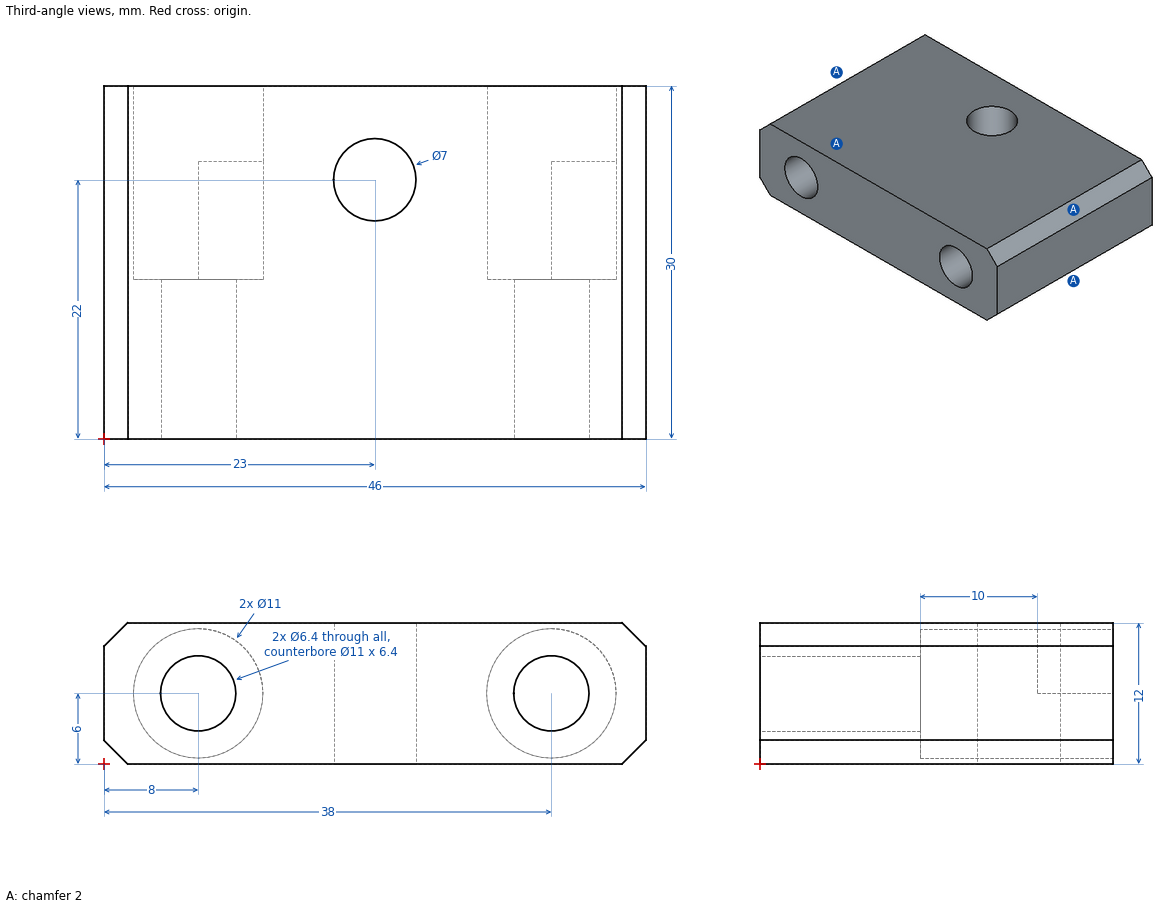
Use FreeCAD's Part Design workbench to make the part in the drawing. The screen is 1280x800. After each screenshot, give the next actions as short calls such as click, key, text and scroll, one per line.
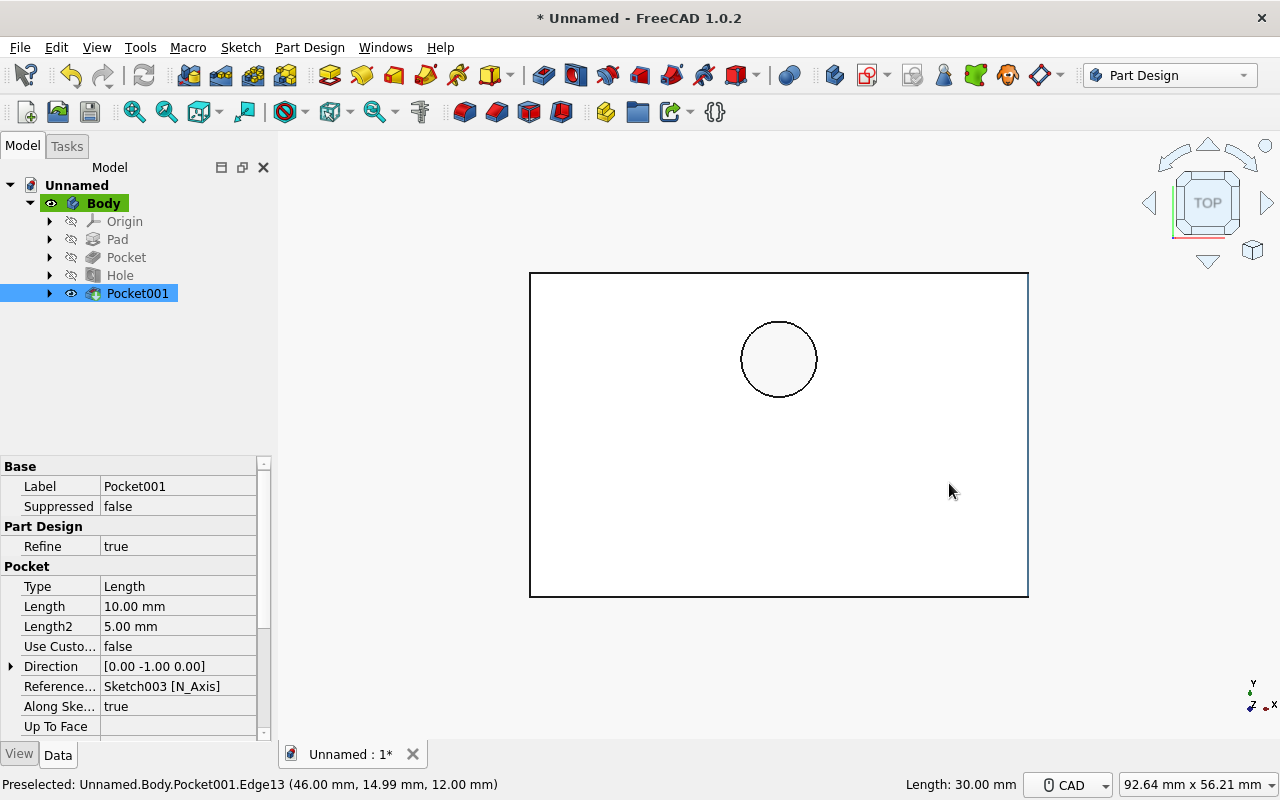
click(530, 434, ctrl)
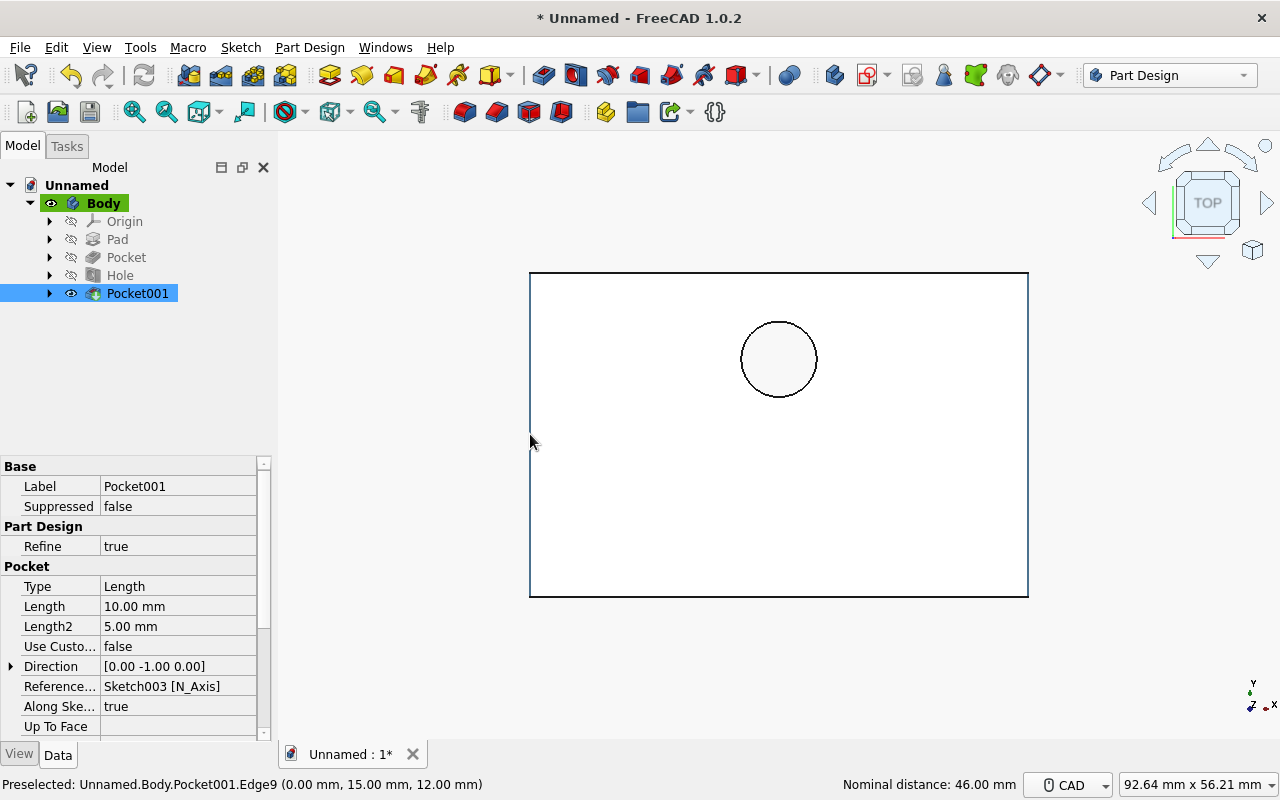
key(1)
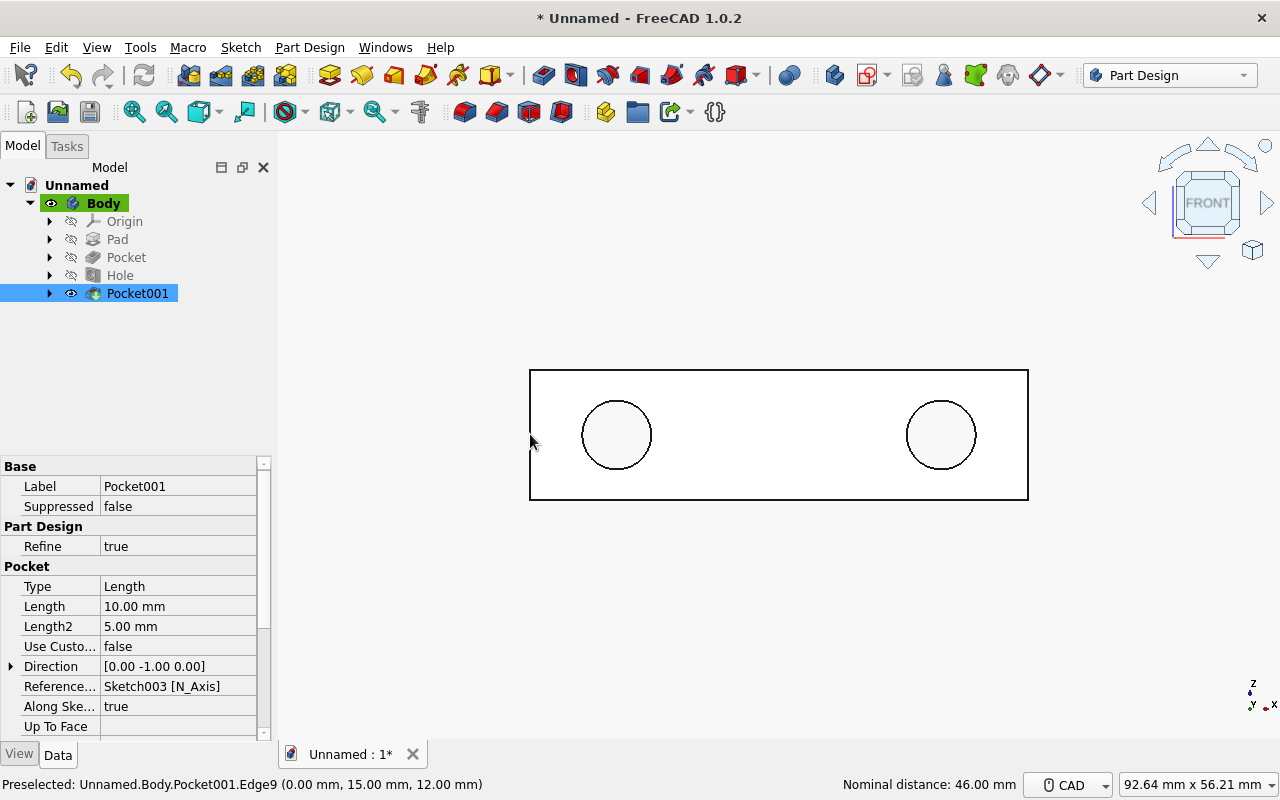
key(3)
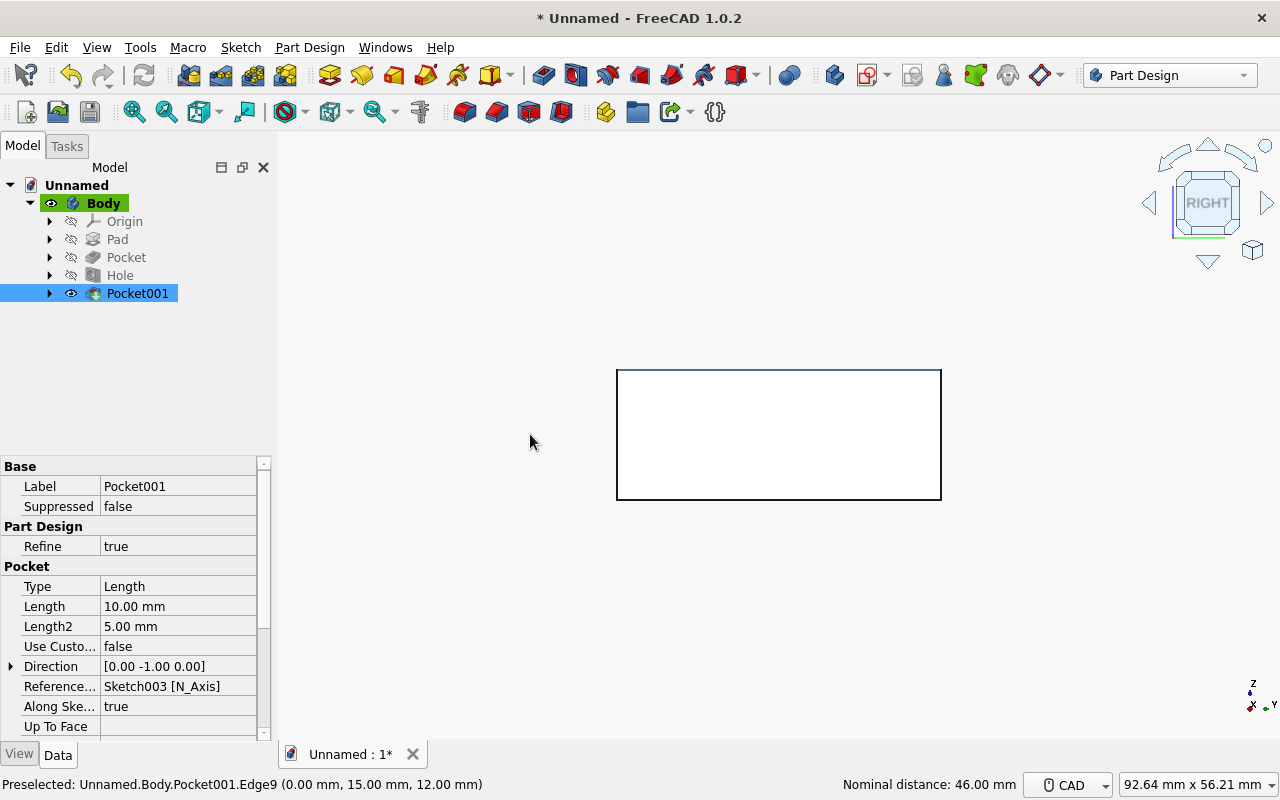
click(136, 112)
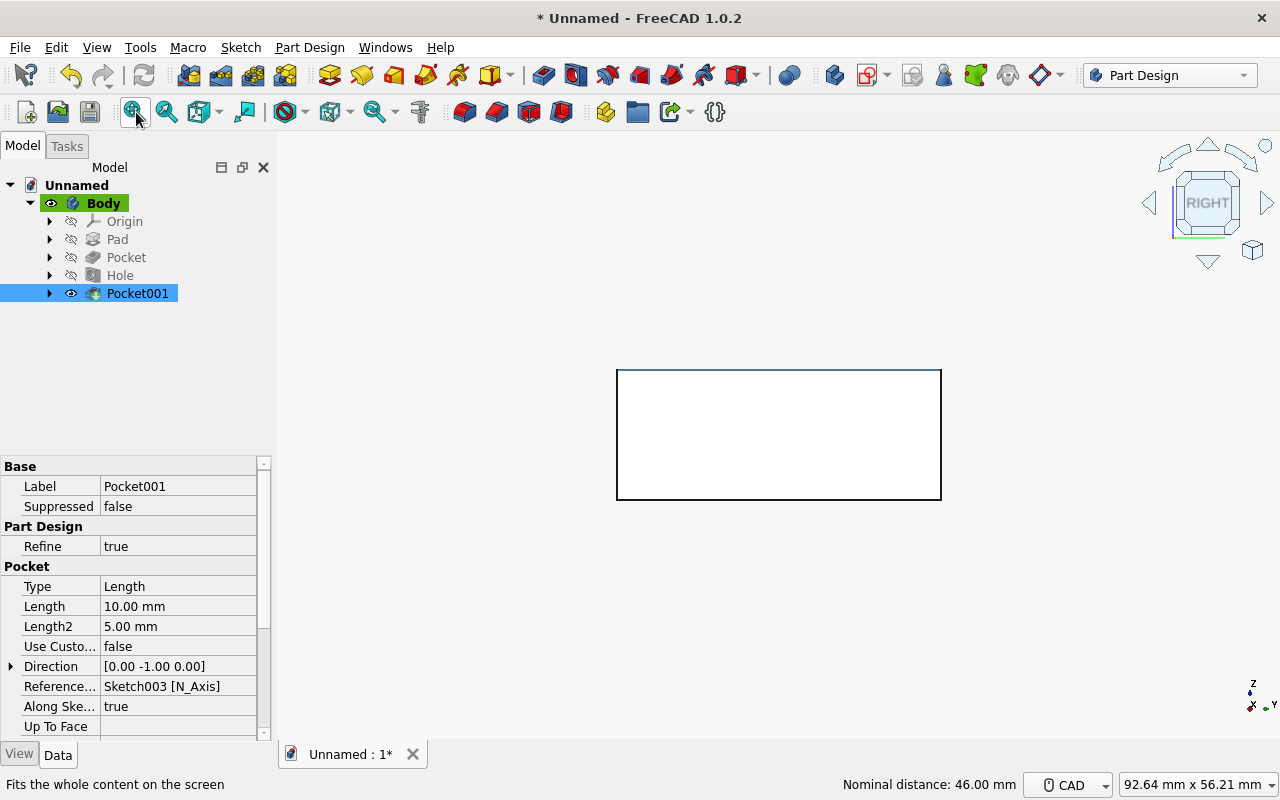
click(779, 499, ctrl)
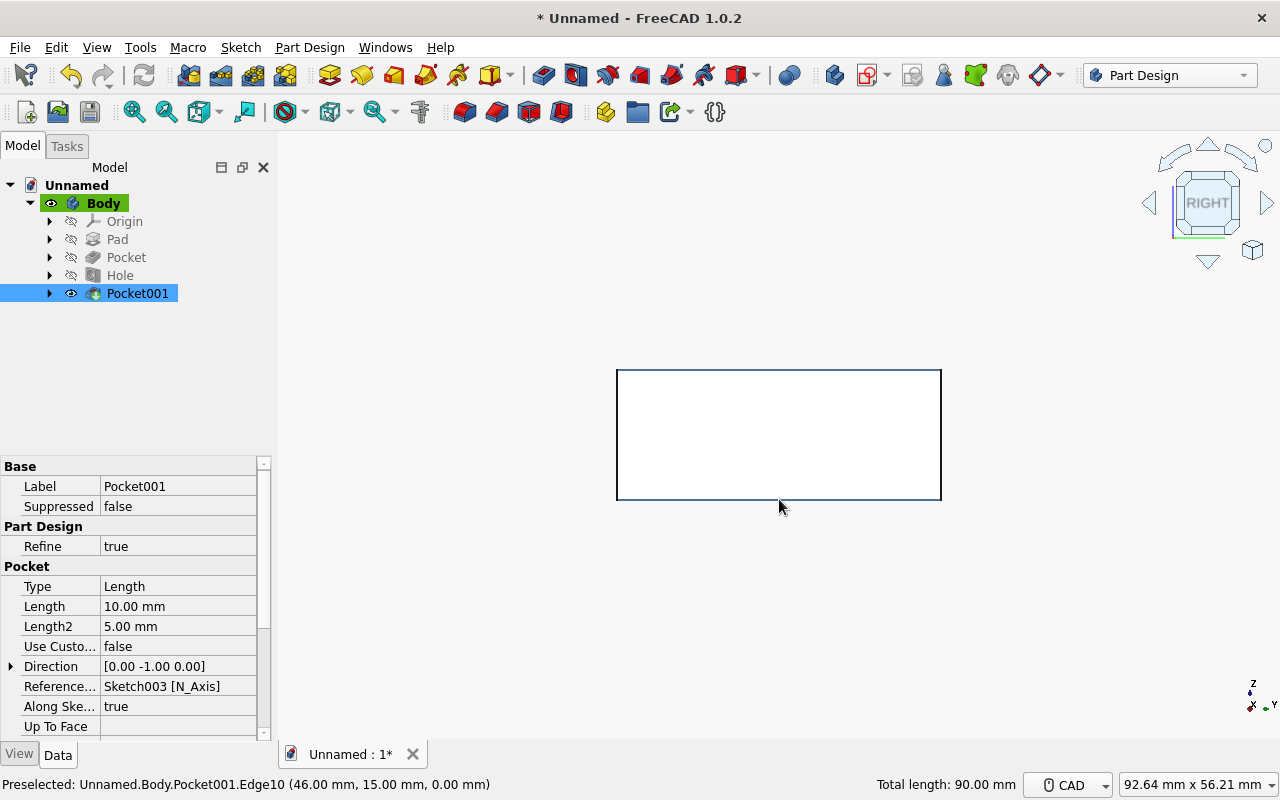
key(5)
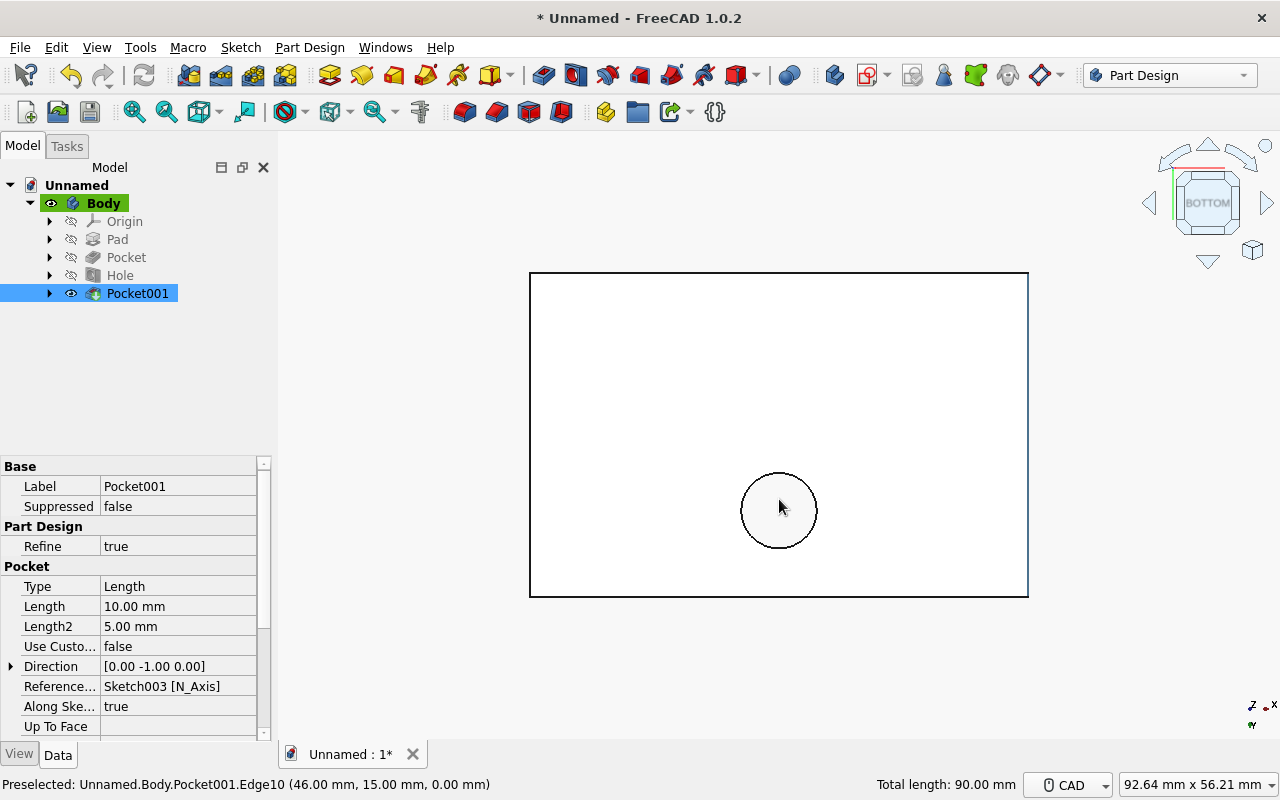
click(530, 434, ctrl)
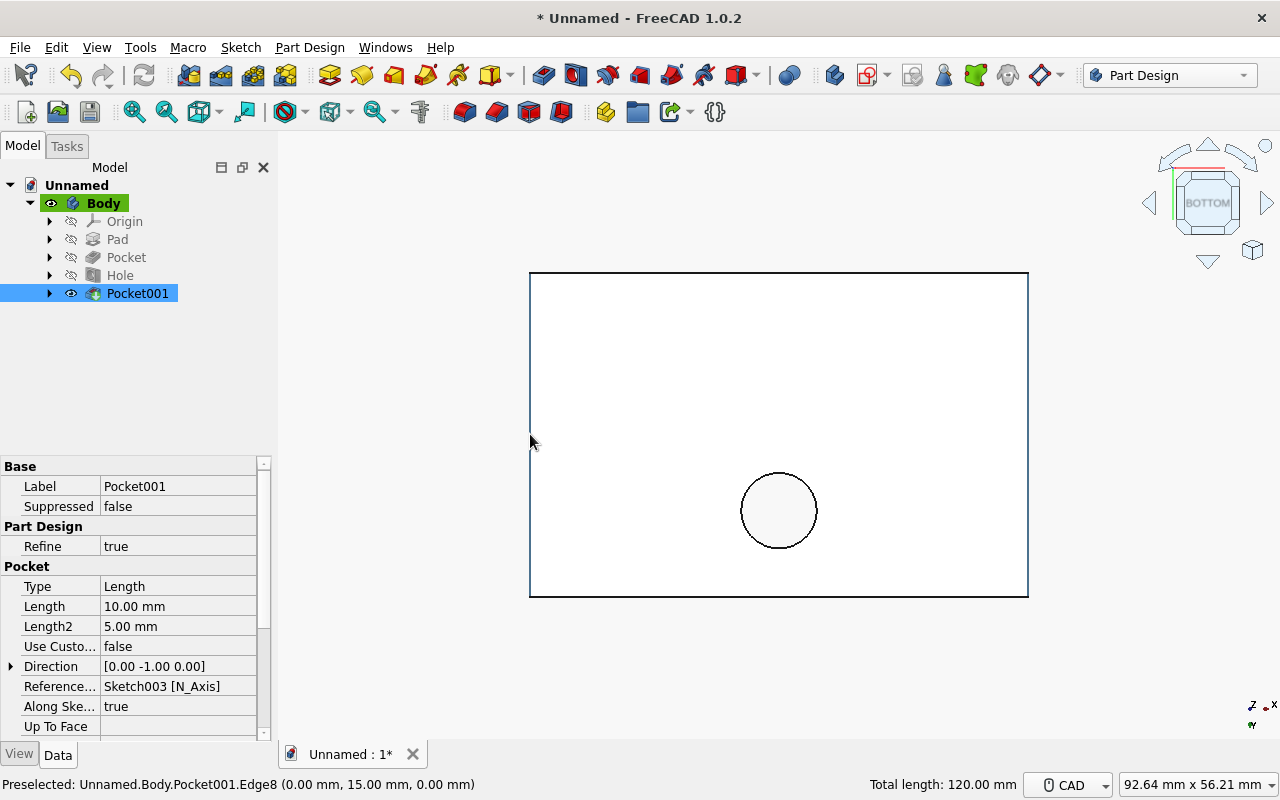
click(498, 112)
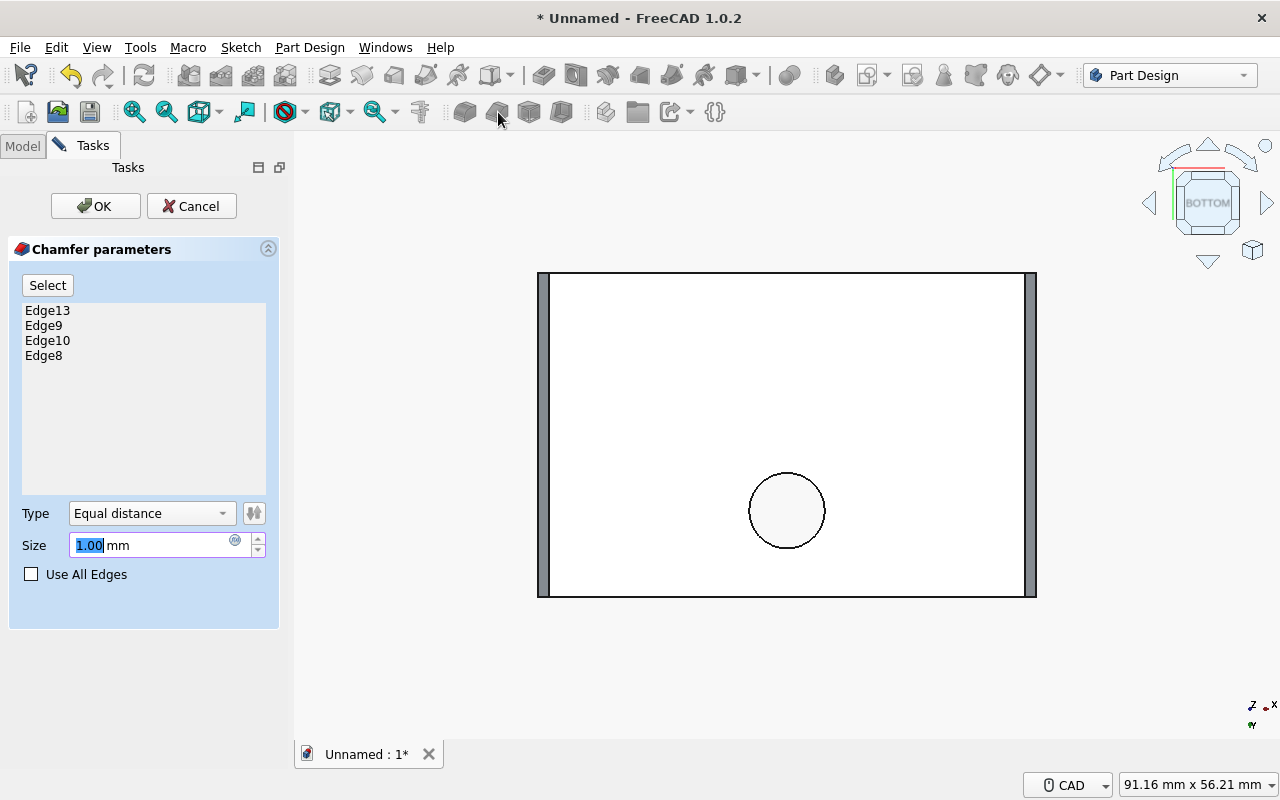
text(2)
key(Tab)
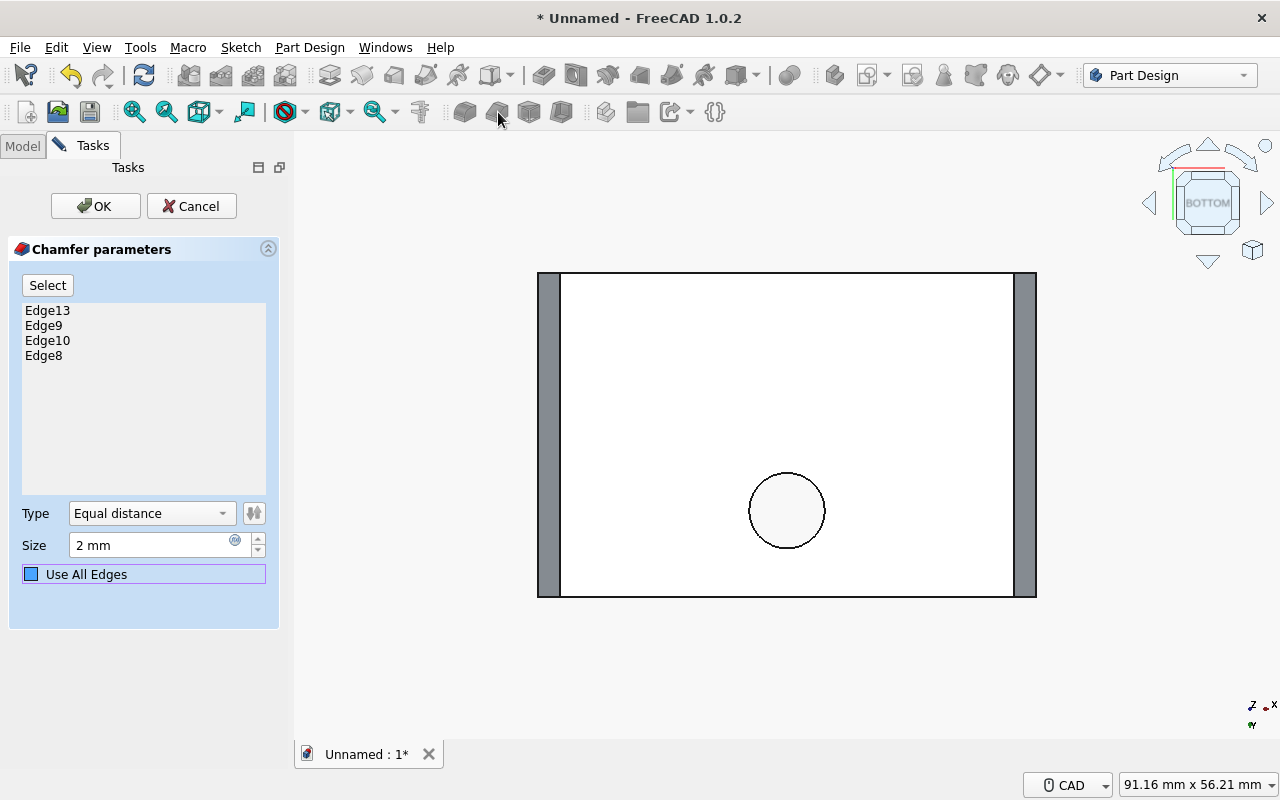
click(96, 206)